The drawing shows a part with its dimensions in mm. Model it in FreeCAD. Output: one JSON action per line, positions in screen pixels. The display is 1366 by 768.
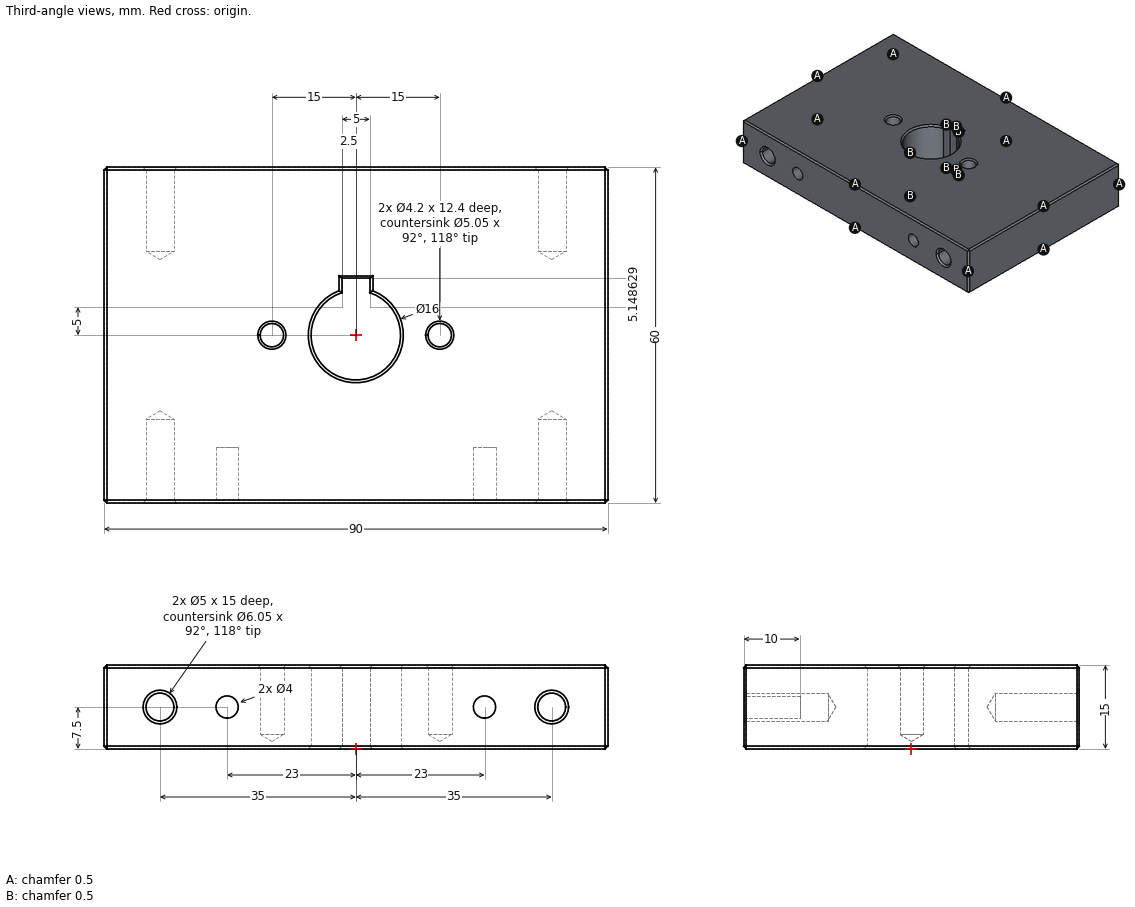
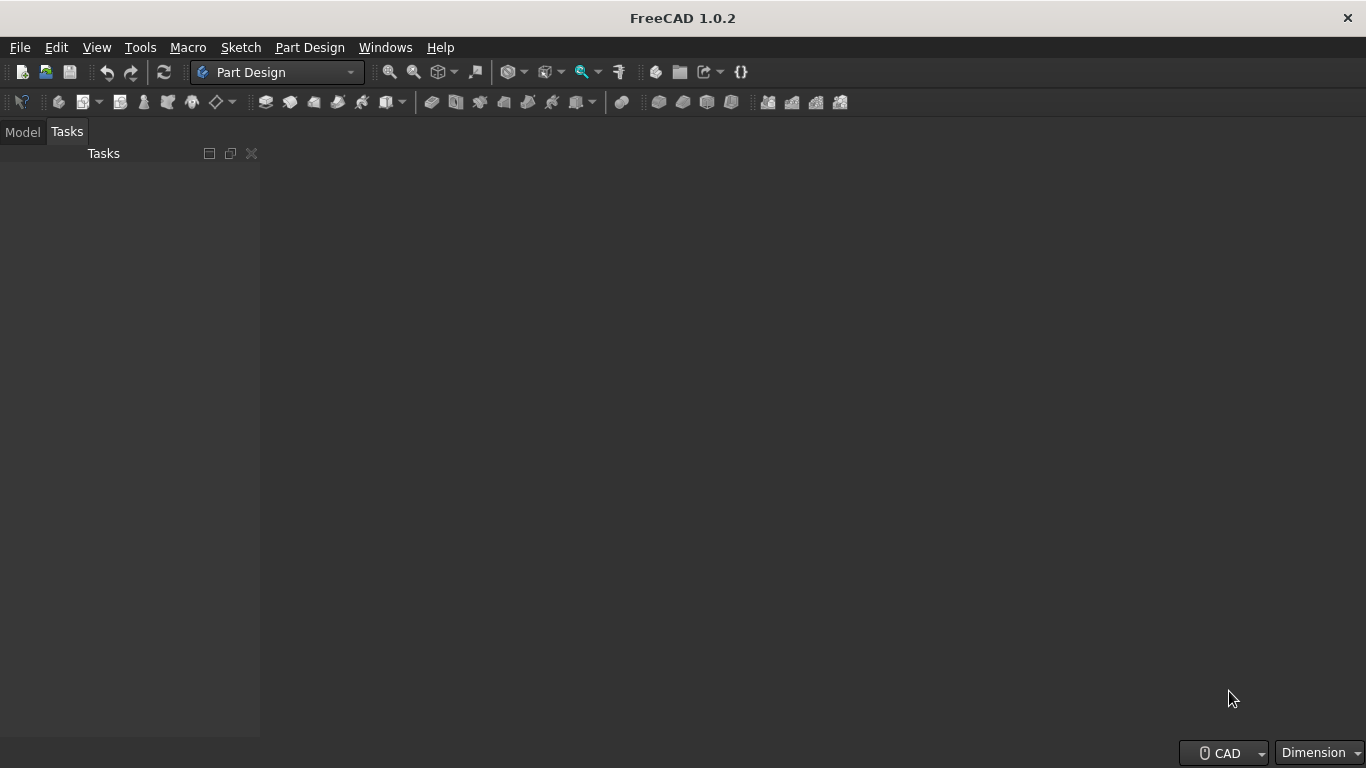
{"action": "key", "text": "ctrl+n"}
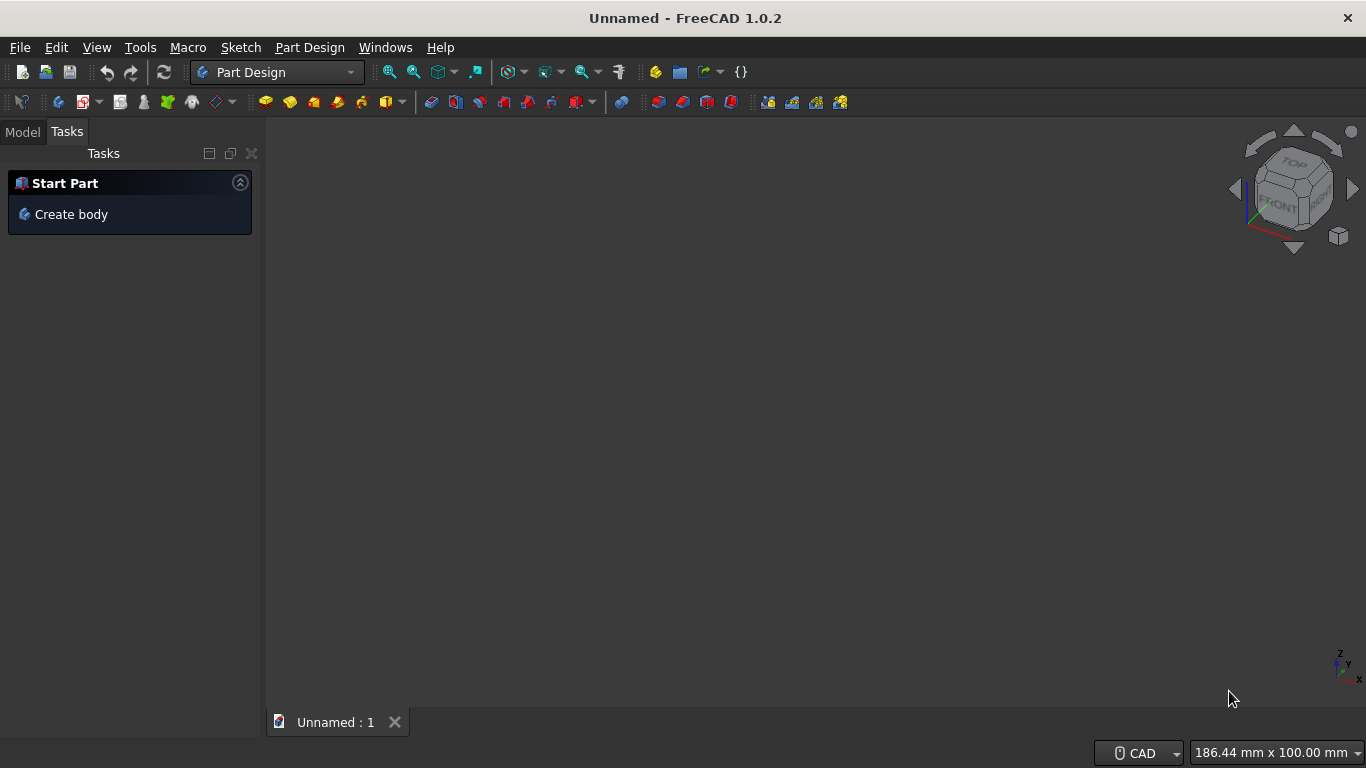
{"action": "left_click", "coordinate": [84, 102]}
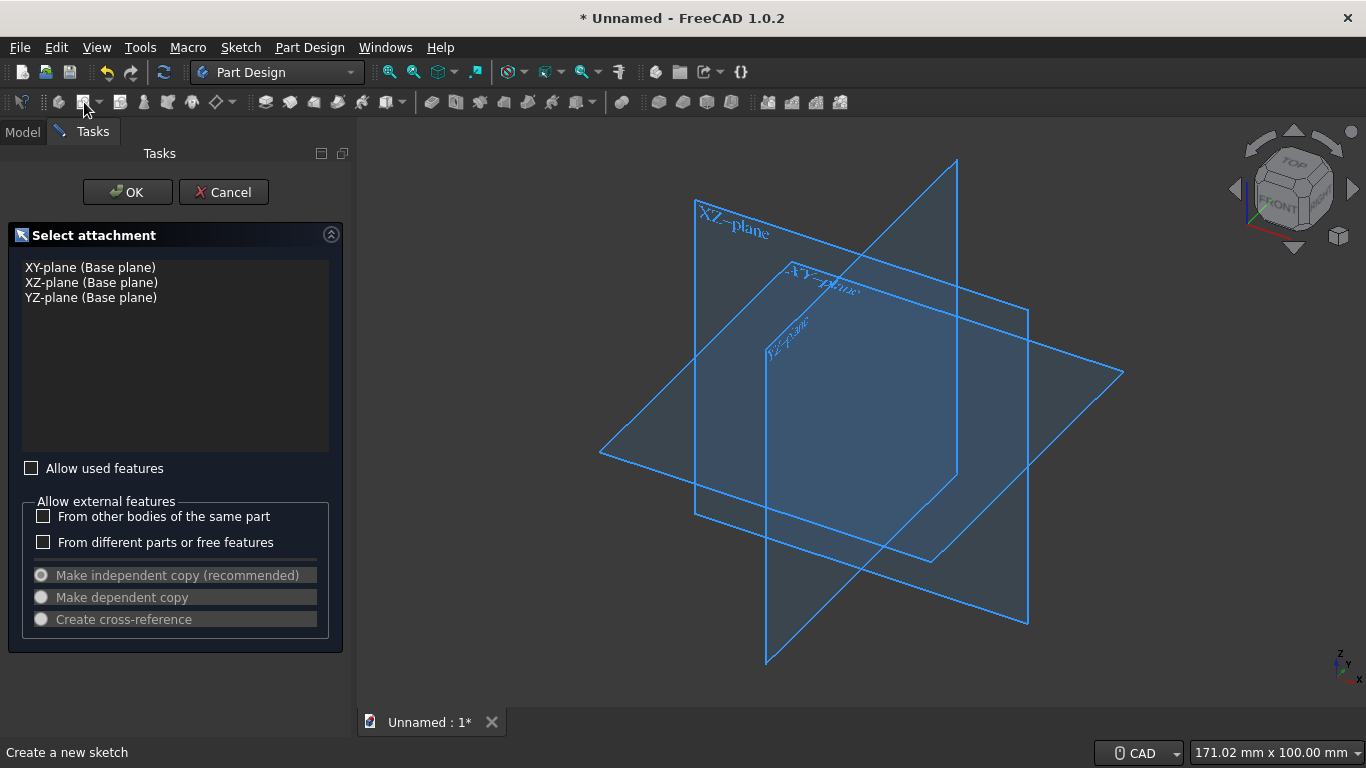
{"action": "left_click", "coordinate": [82, 268]}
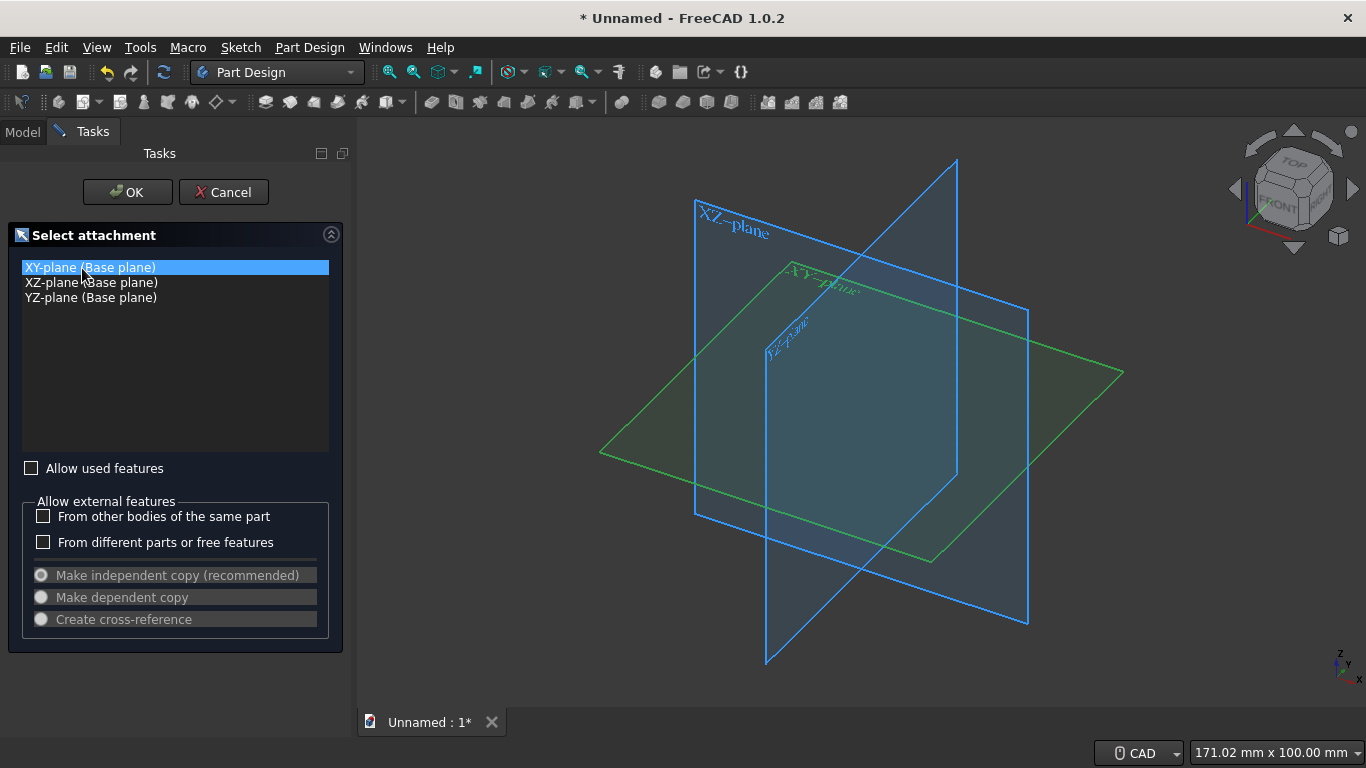
{"action": "left_click", "coordinate": [128, 192]}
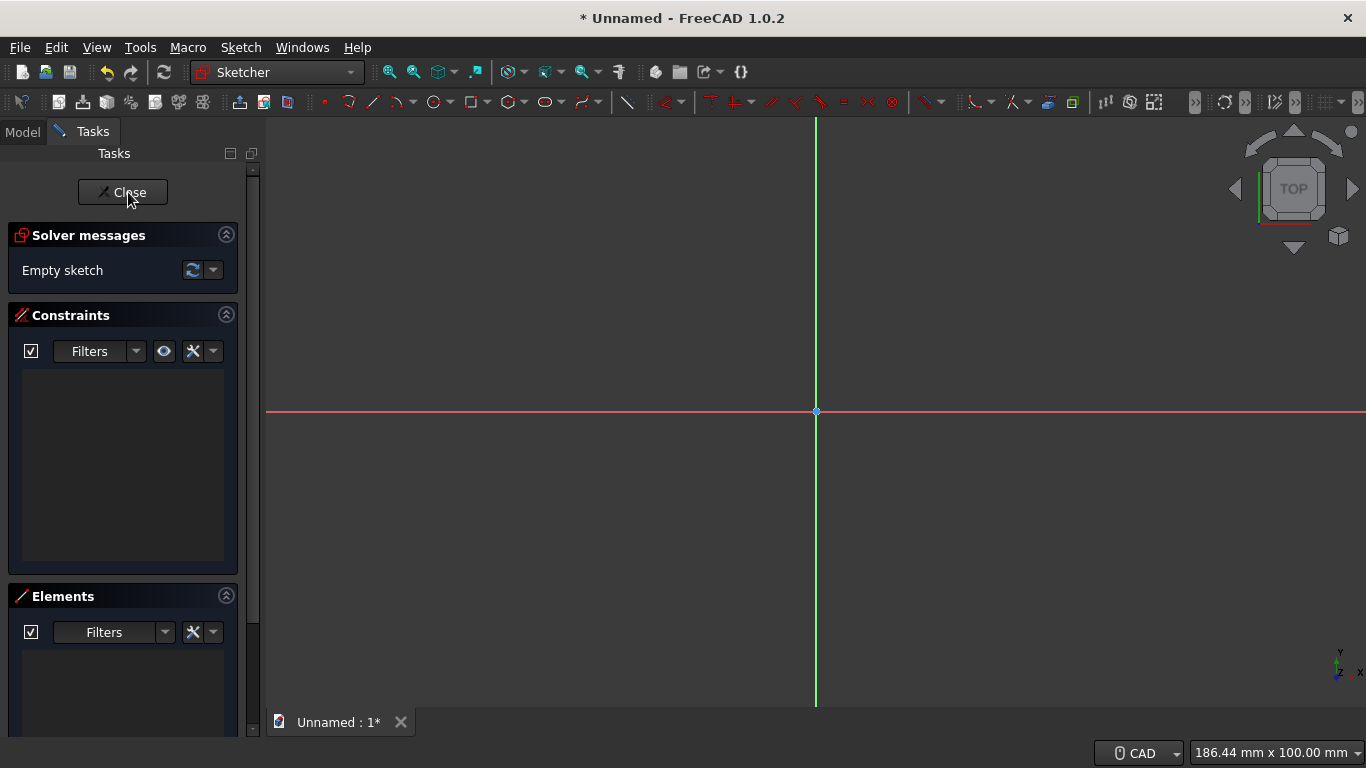
{"action": "key", "text": "g v"}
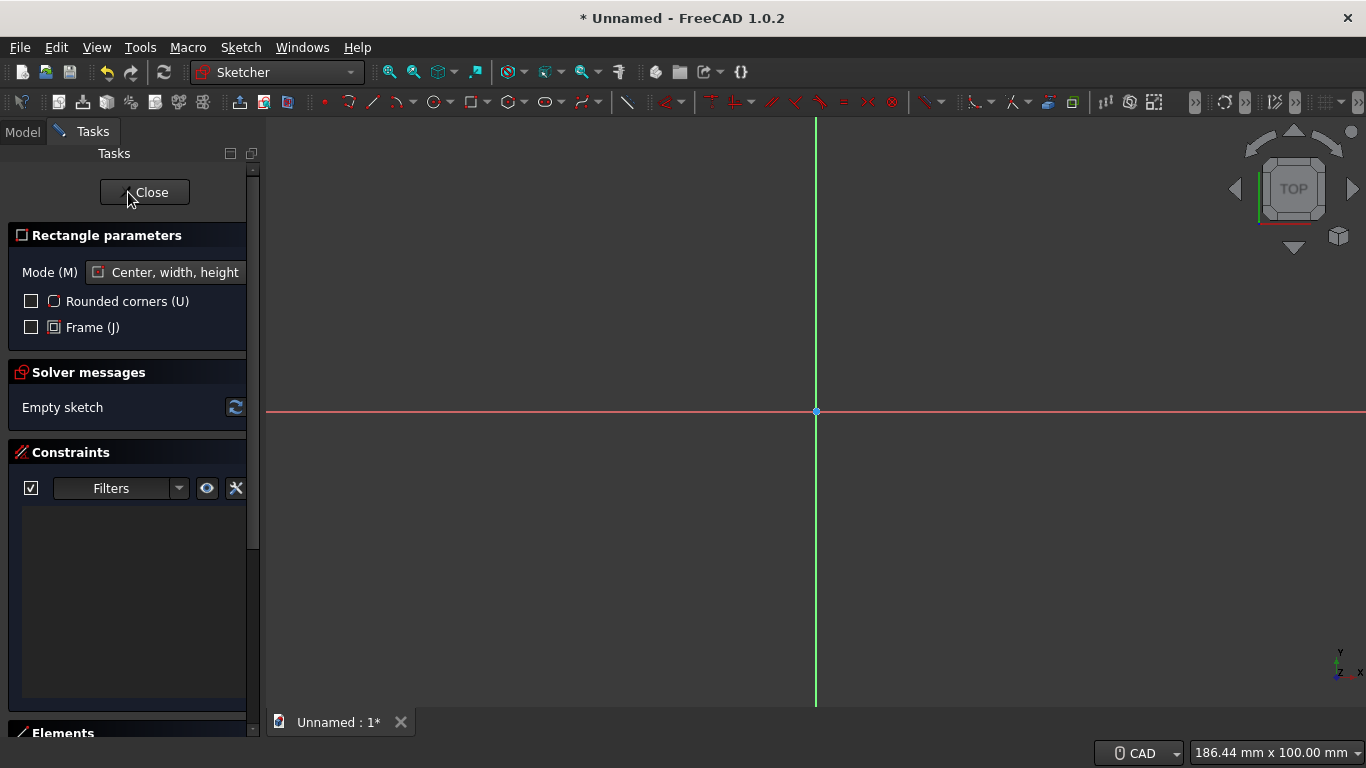
{"action": "left_click", "coordinate": [816, 412]}
{"action": "mouse_move", "coordinate": [1082, 235]}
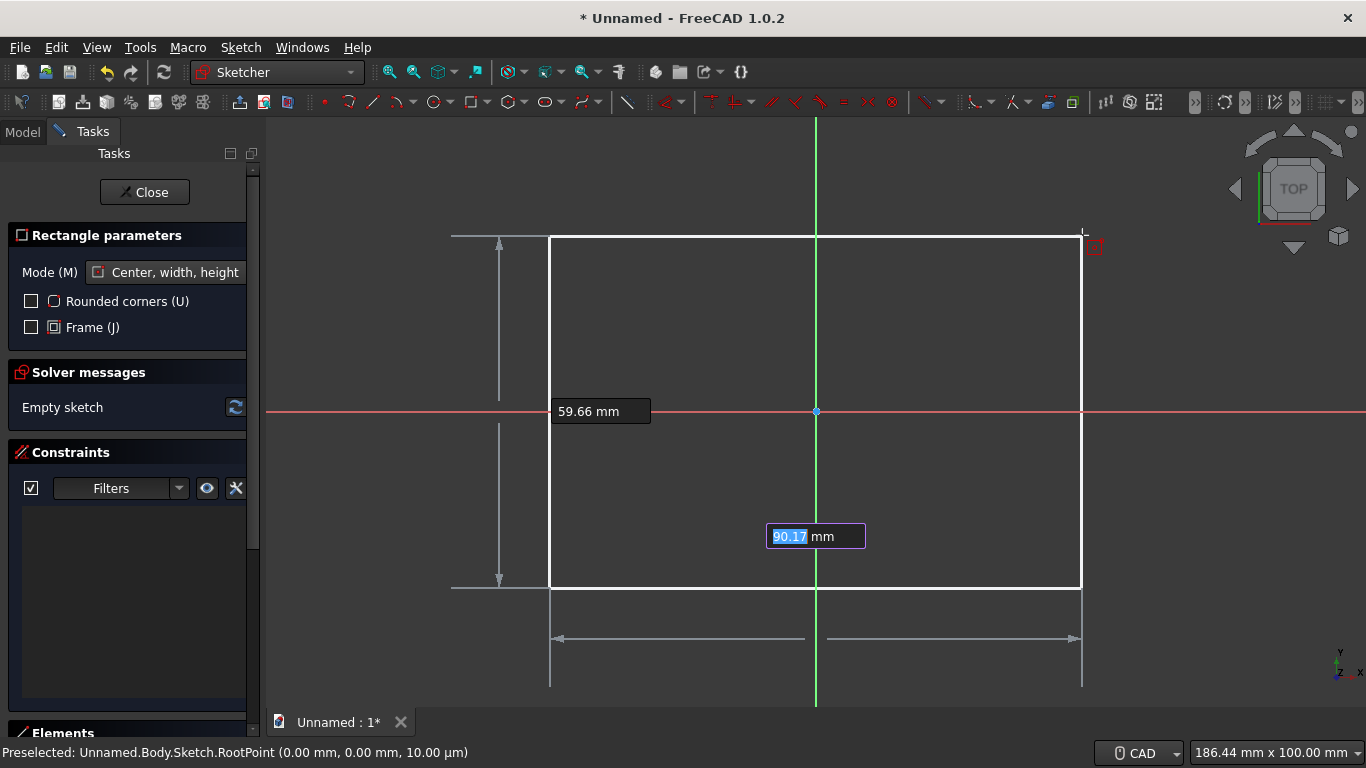
{"action": "type", "text": "90"}
{"action": "key", "text": "Tab"}
{"action": "type", "text": "60"}
{"action": "key", "text": "Return"}
{"action": "key", "text": "Escape"}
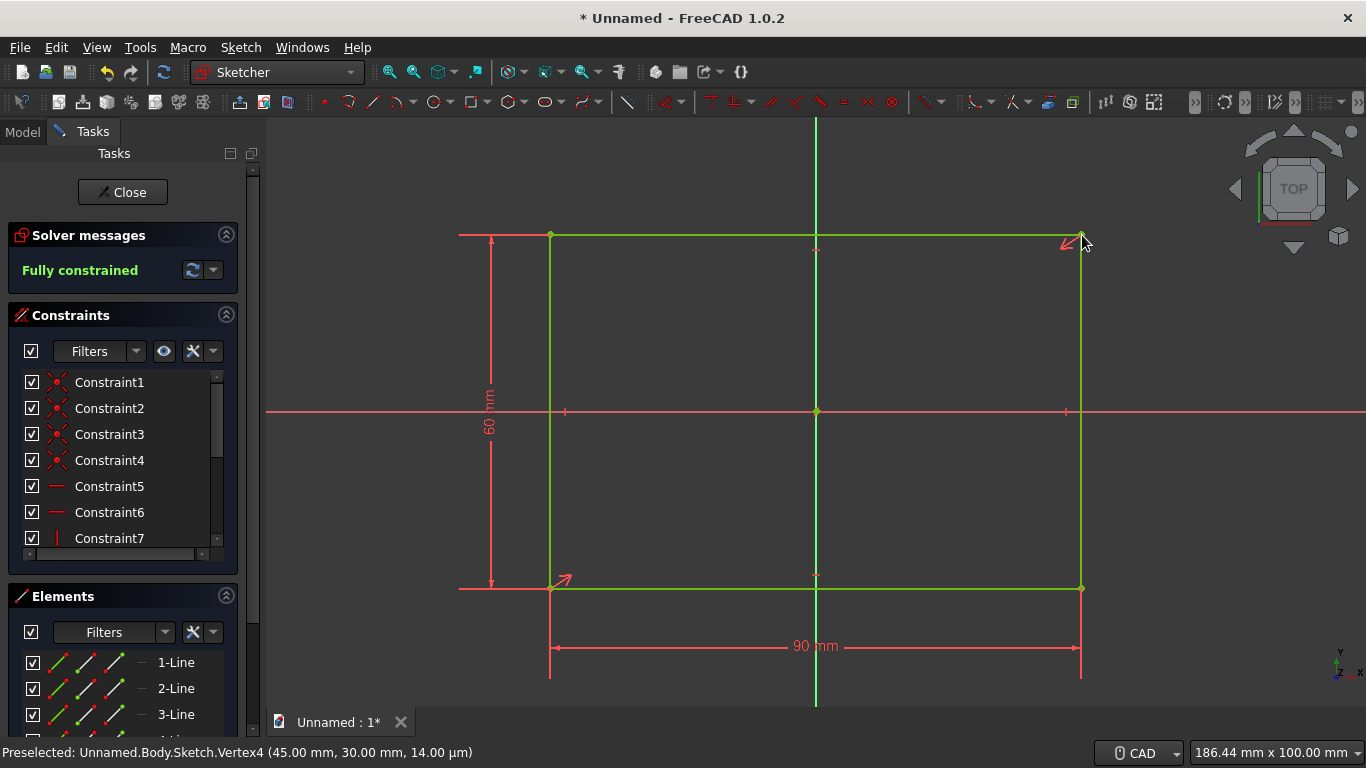
{"action": "left_click", "coordinate": [123, 192]}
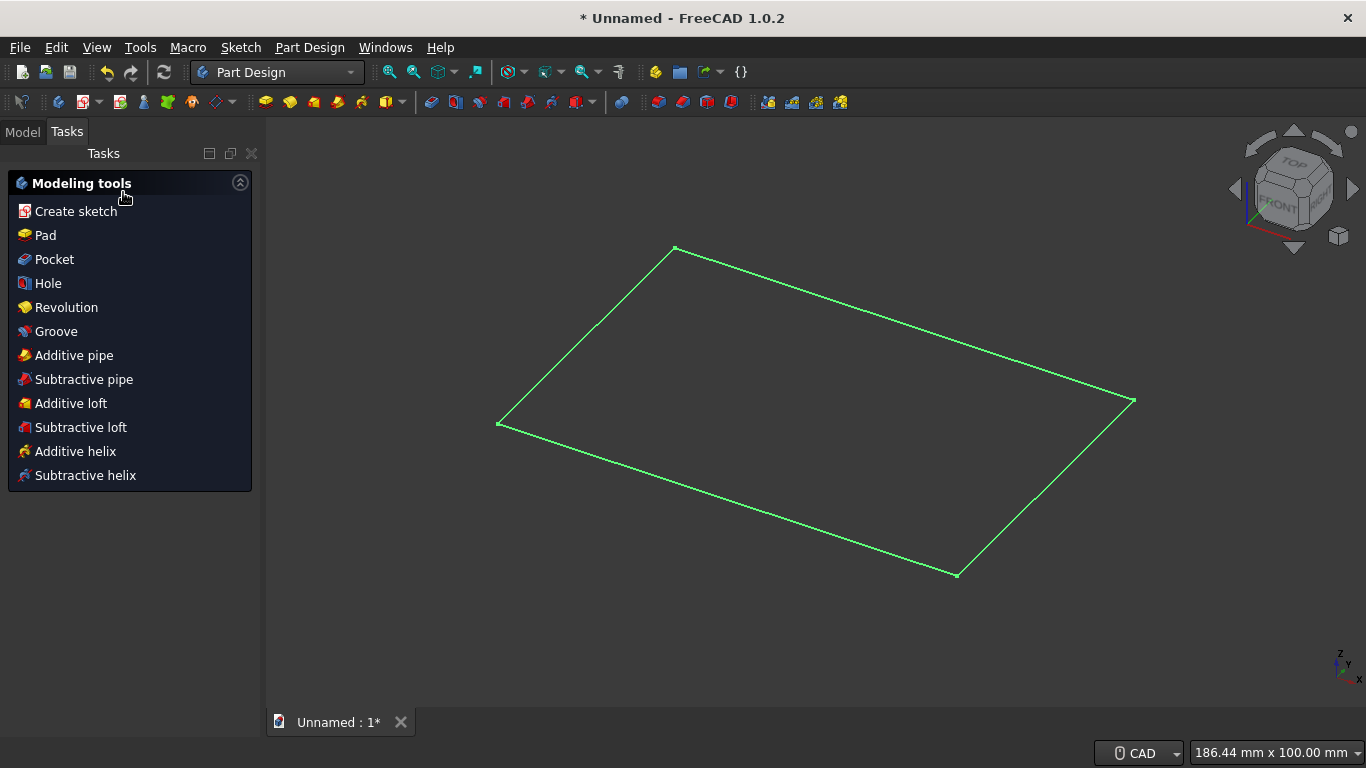
{"action": "left_click", "coordinate": [266, 102]}